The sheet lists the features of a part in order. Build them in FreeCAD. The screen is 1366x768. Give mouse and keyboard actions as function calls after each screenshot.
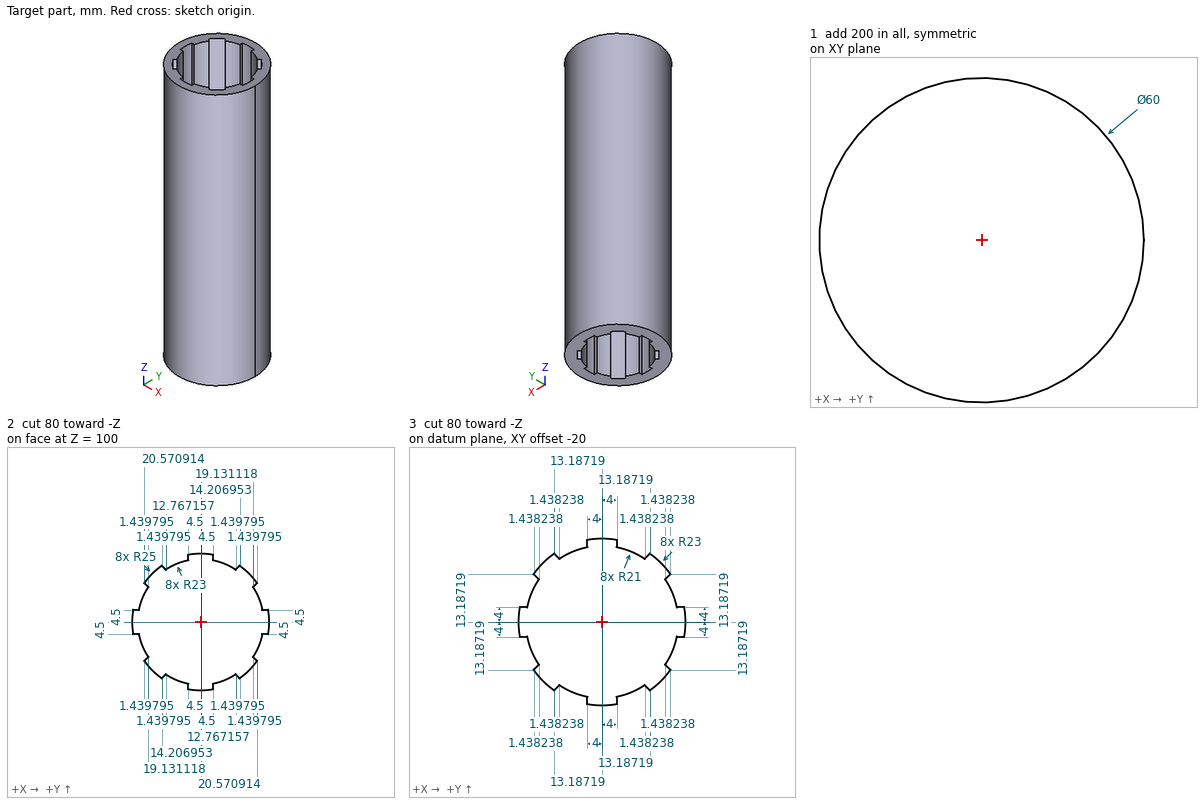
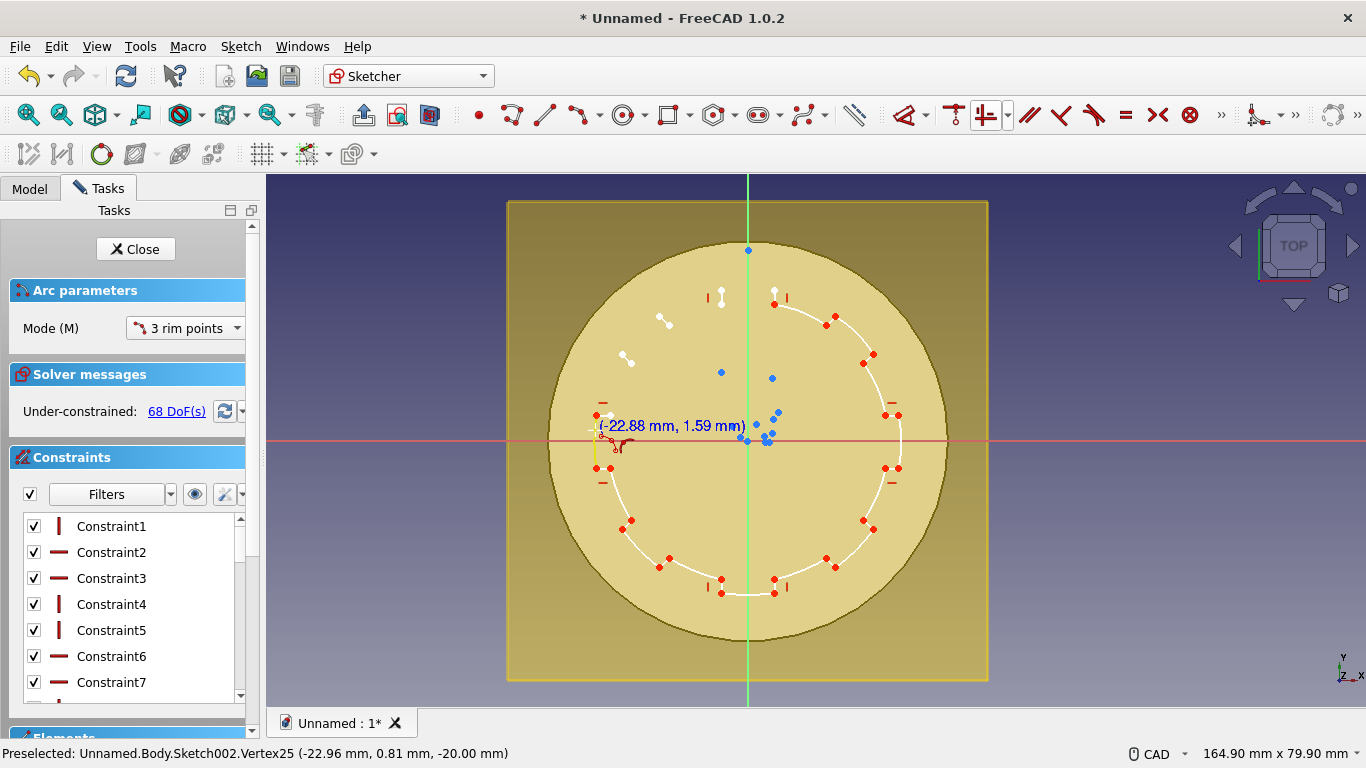
scroll(610, 414, up, 5)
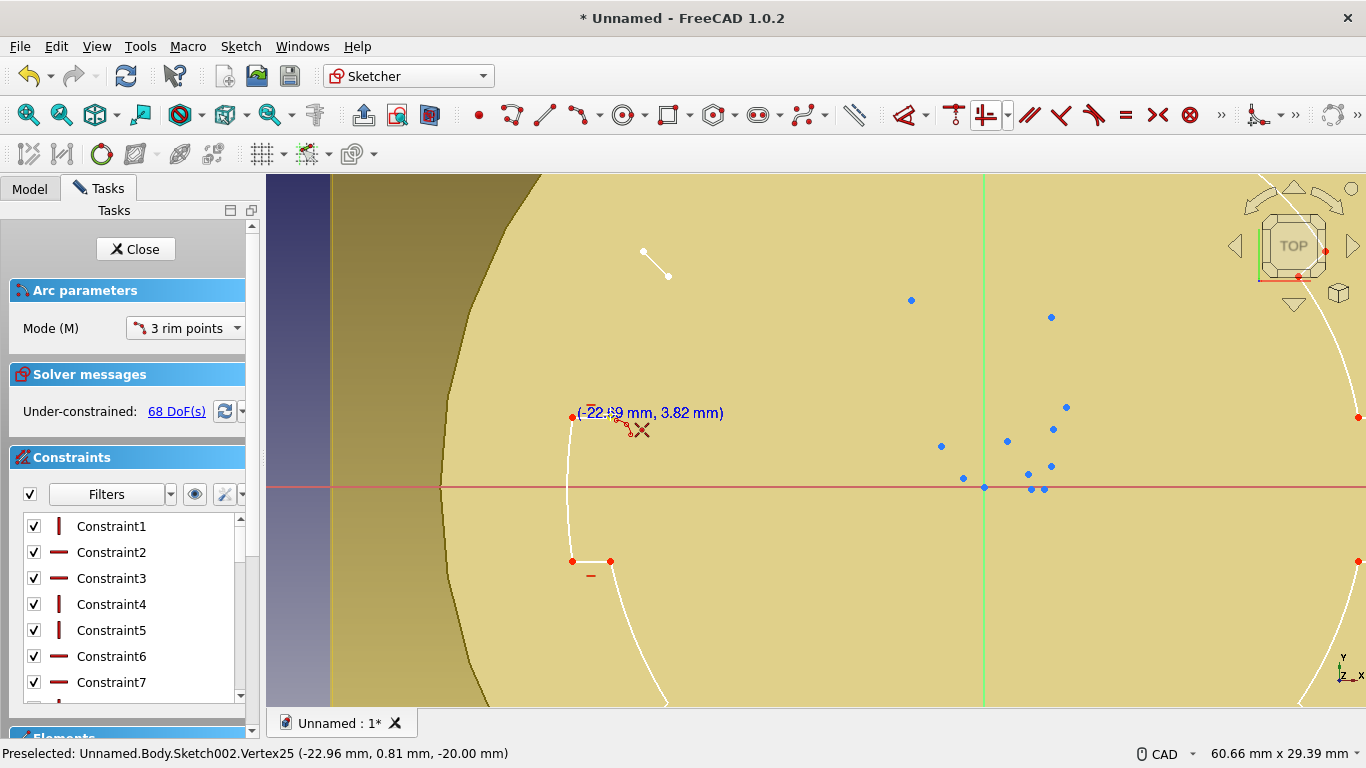
click(611, 418)
click(668, 276)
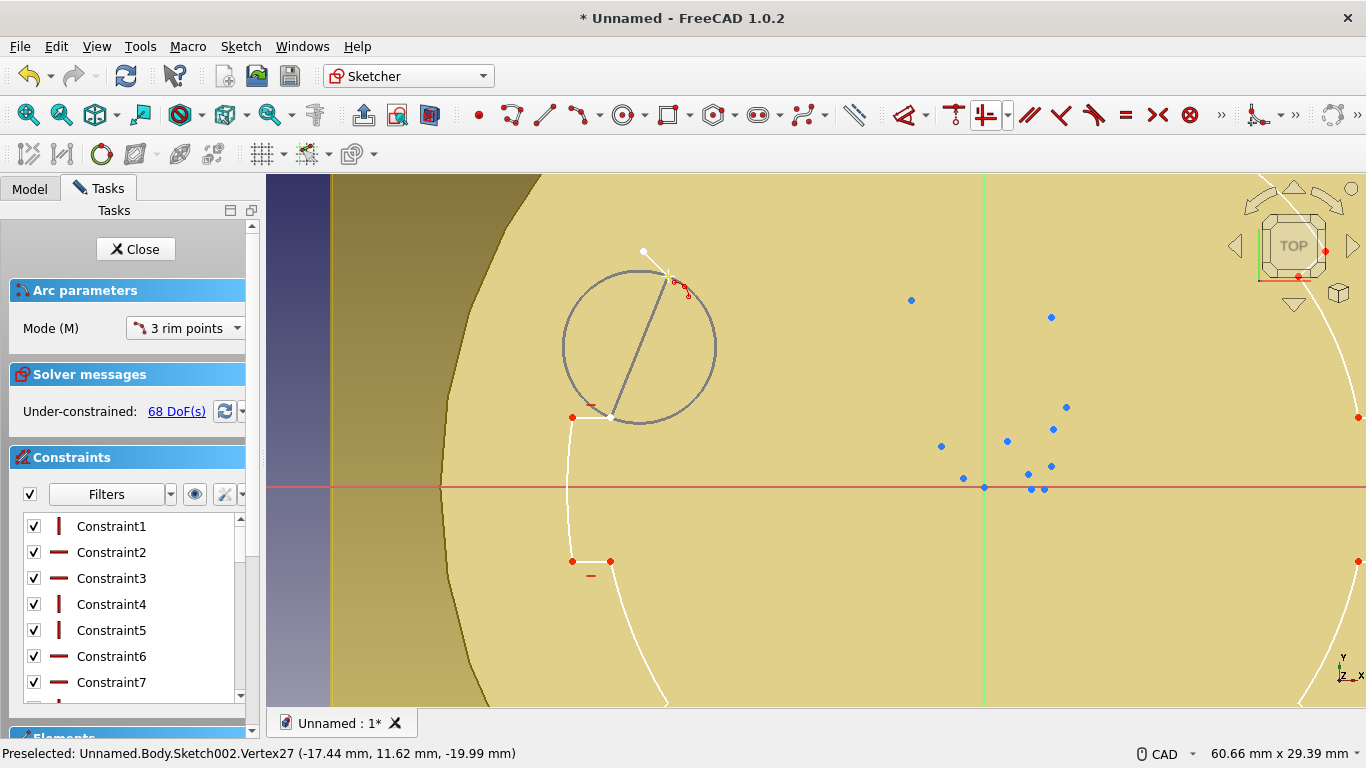
scroll(632, 341, up, 4)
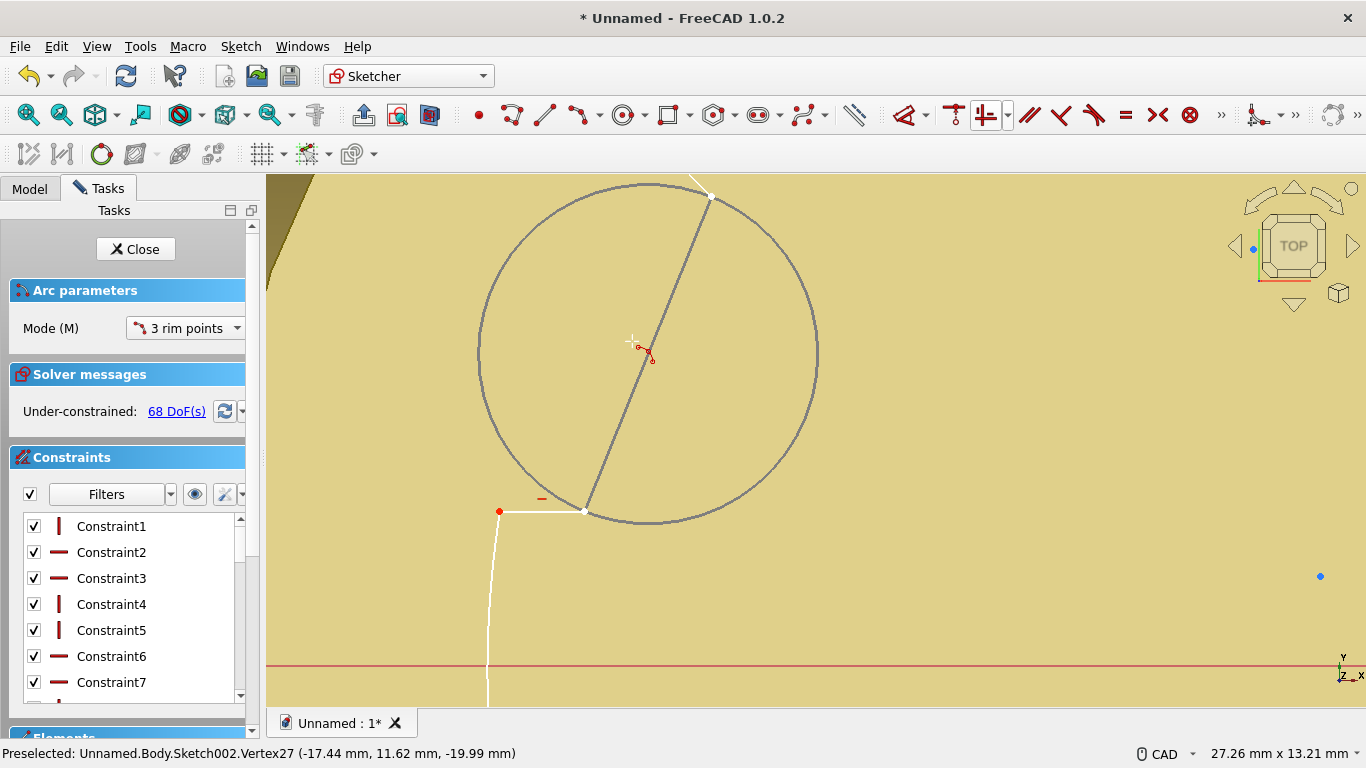
click(633, 341)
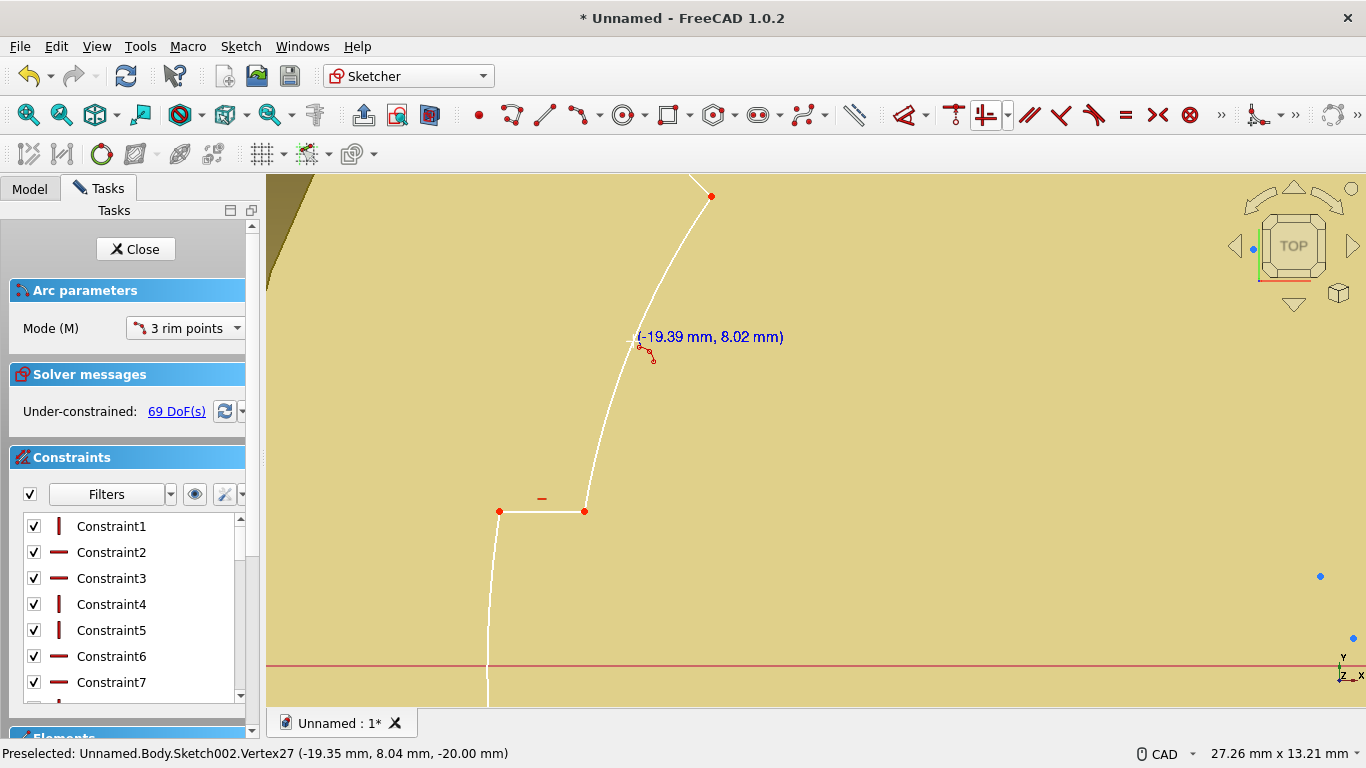
scroll(615, 396, down, 9)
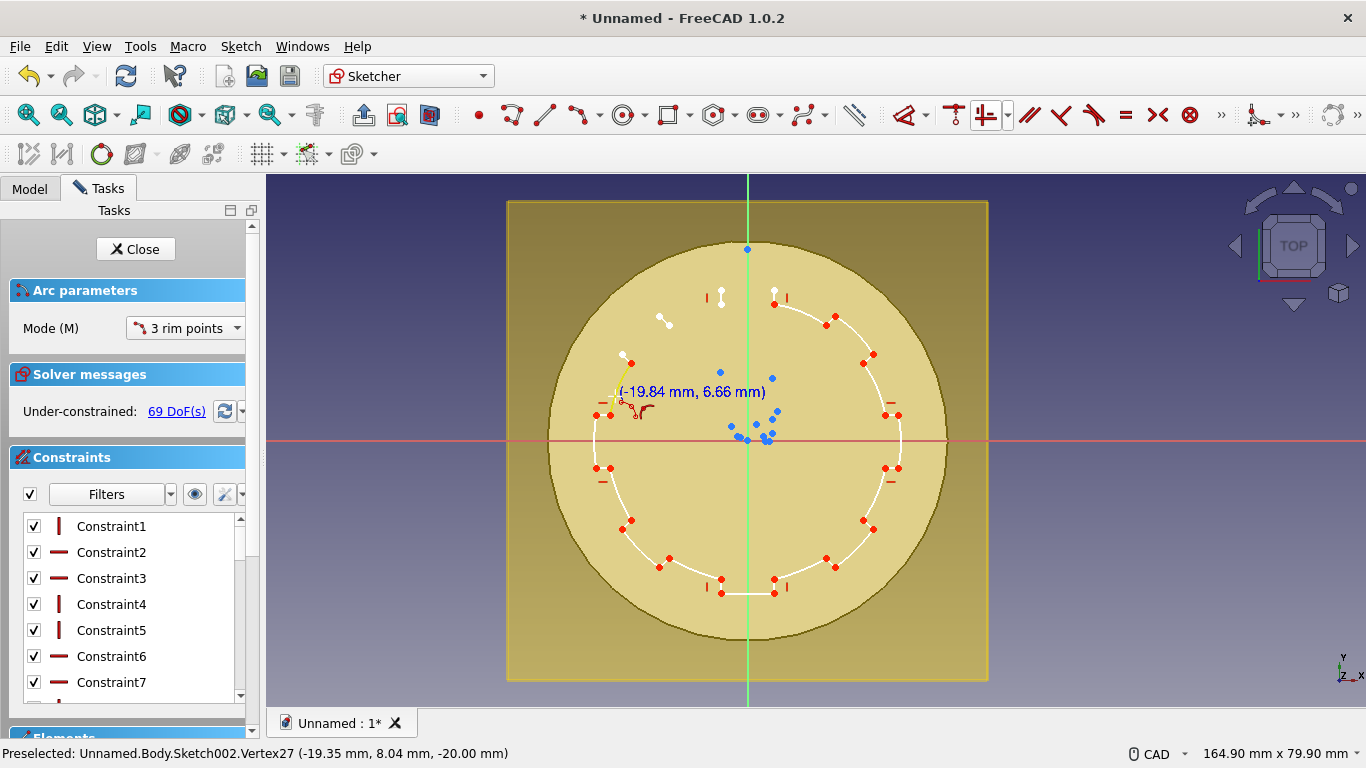
scroll(622, 353, up, 5)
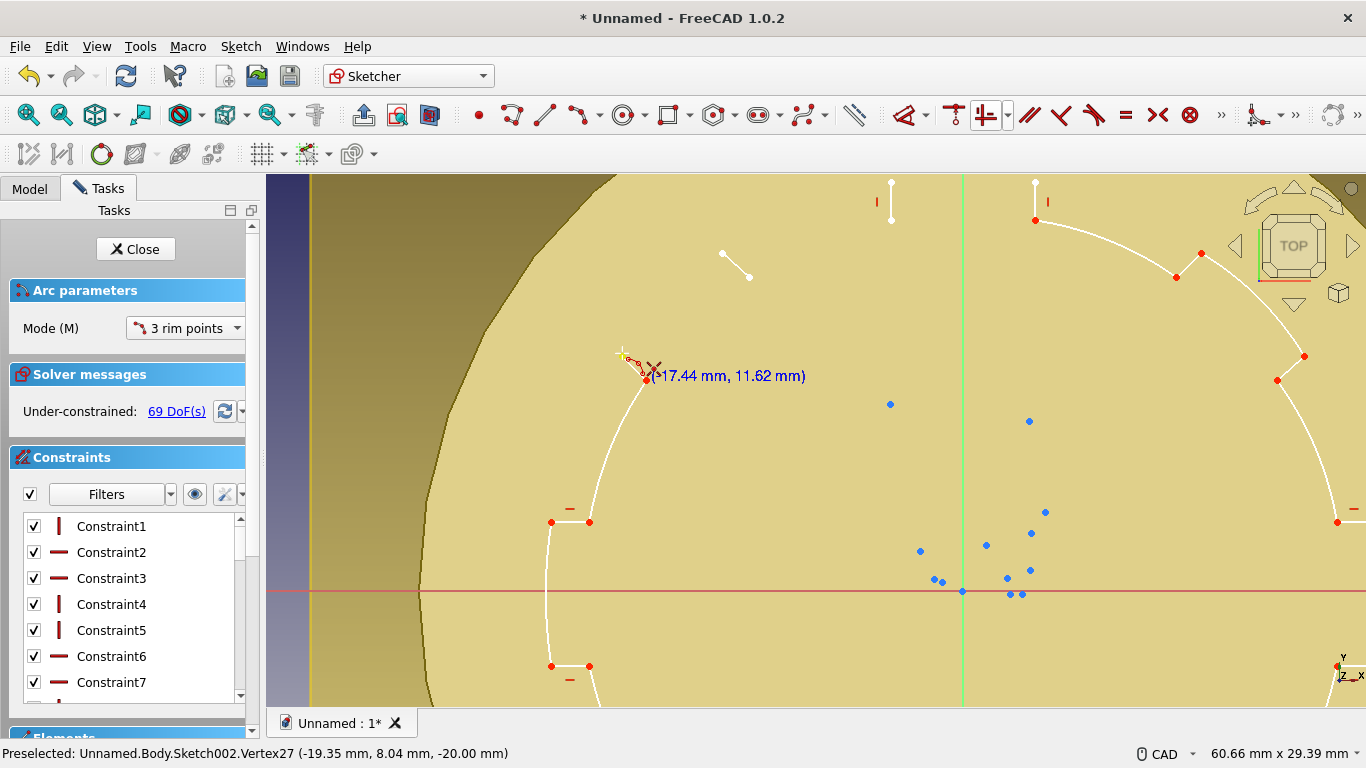
click(622, 356)
click(723, 253)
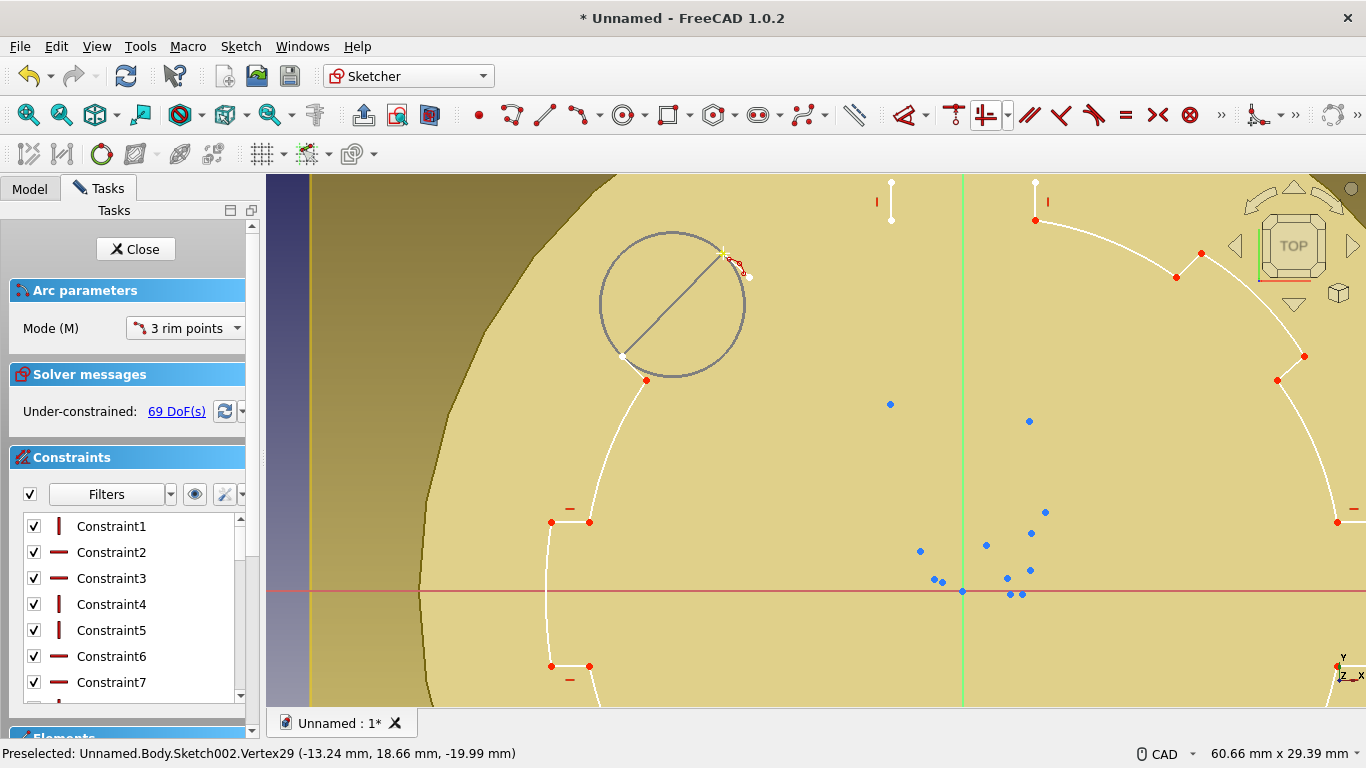
scroll(668, 297, up, 5)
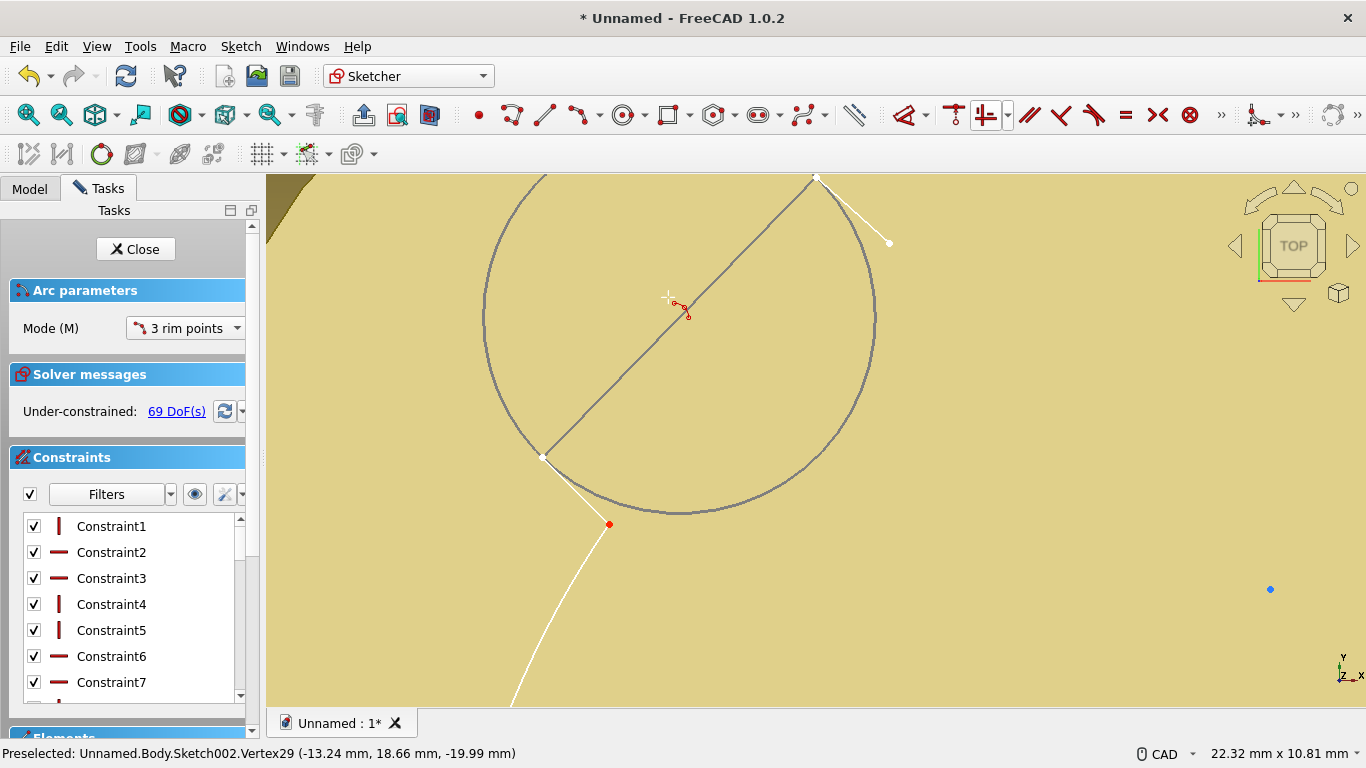
click(667, 295)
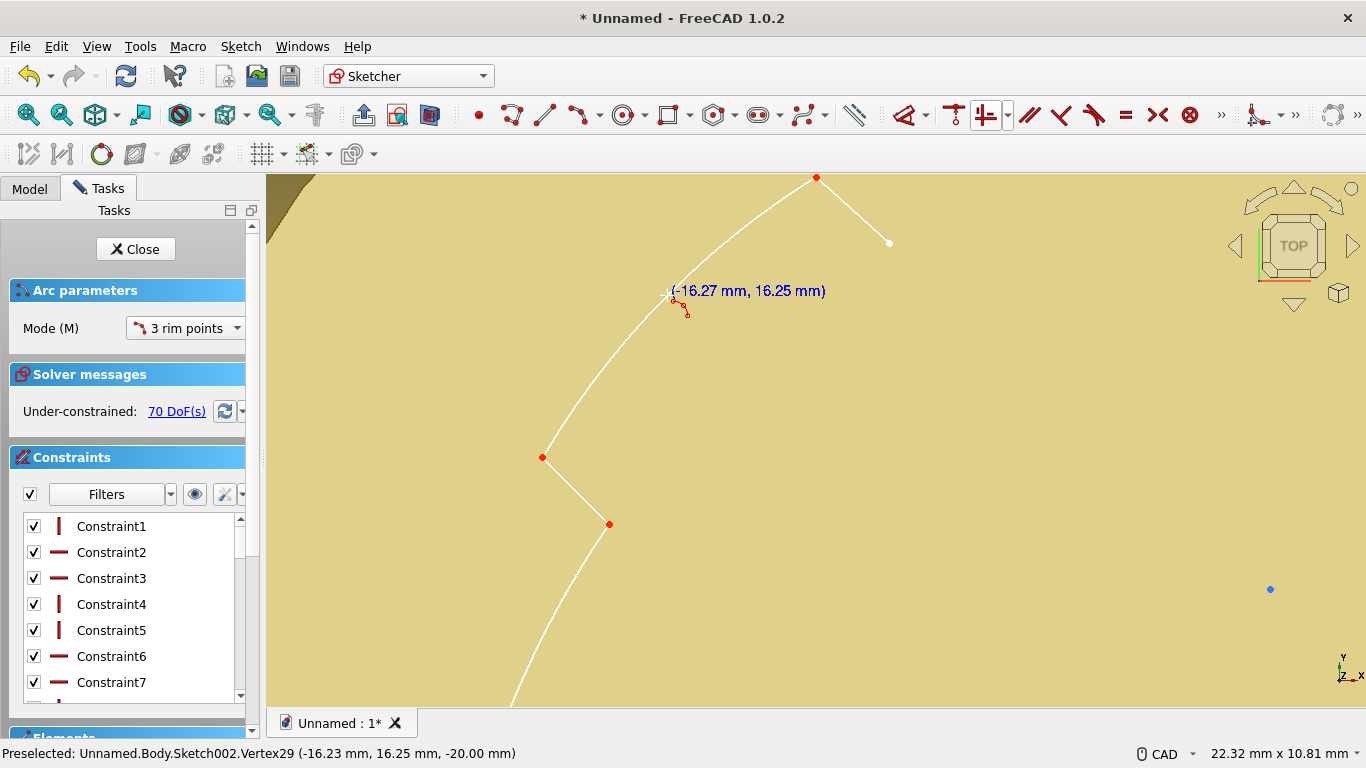
scroll(635, 338, down, 10)